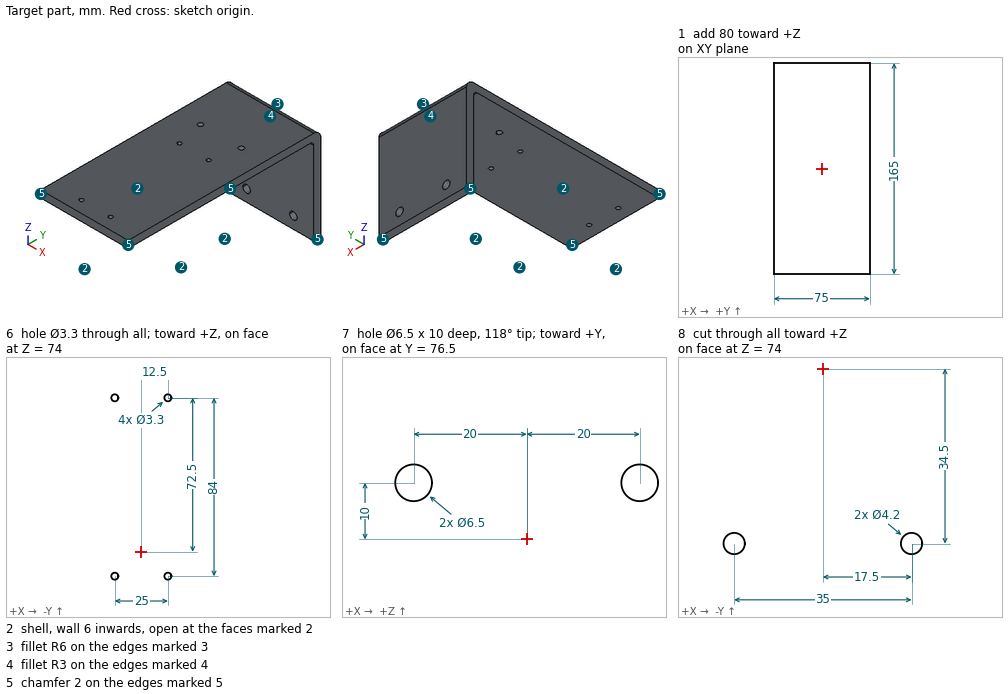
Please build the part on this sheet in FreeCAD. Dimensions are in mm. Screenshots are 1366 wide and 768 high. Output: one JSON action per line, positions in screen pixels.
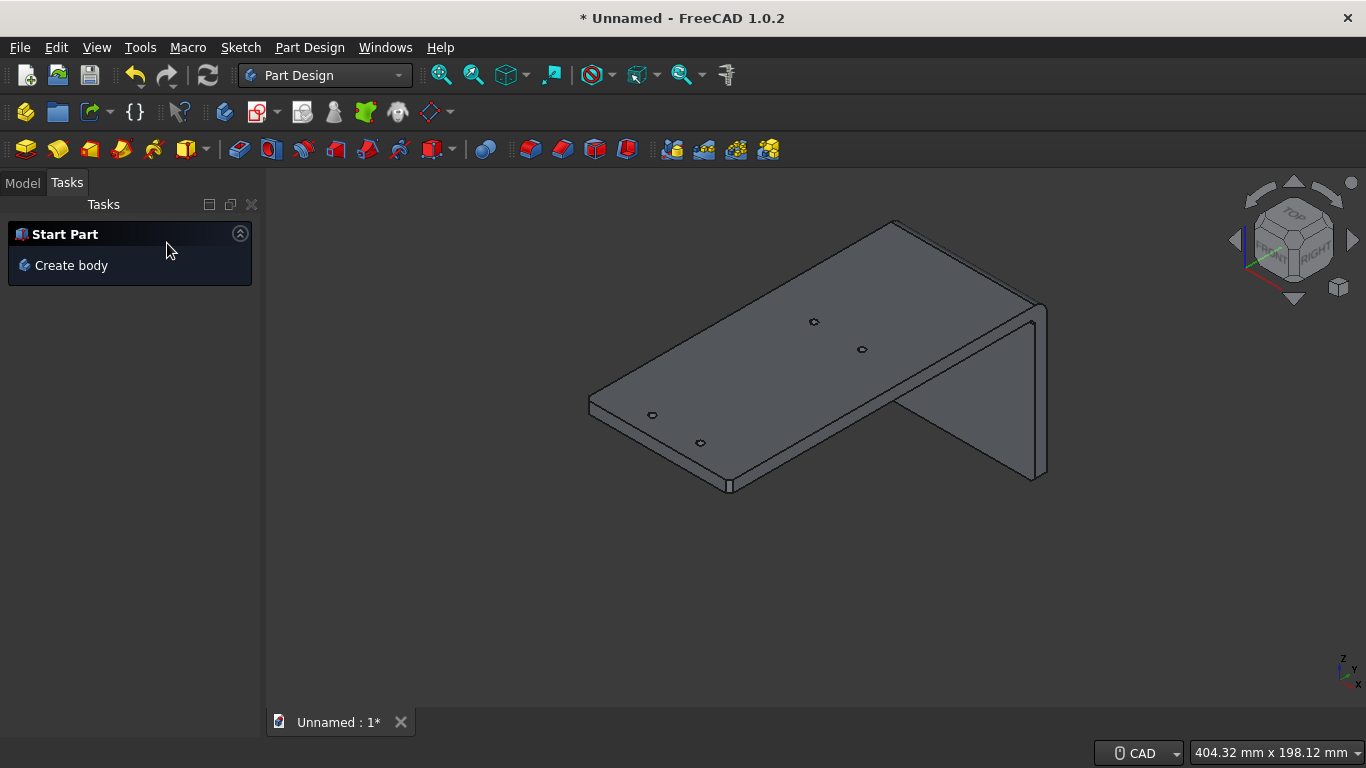
{"action": "left_click", "coordinate": [984, 373]}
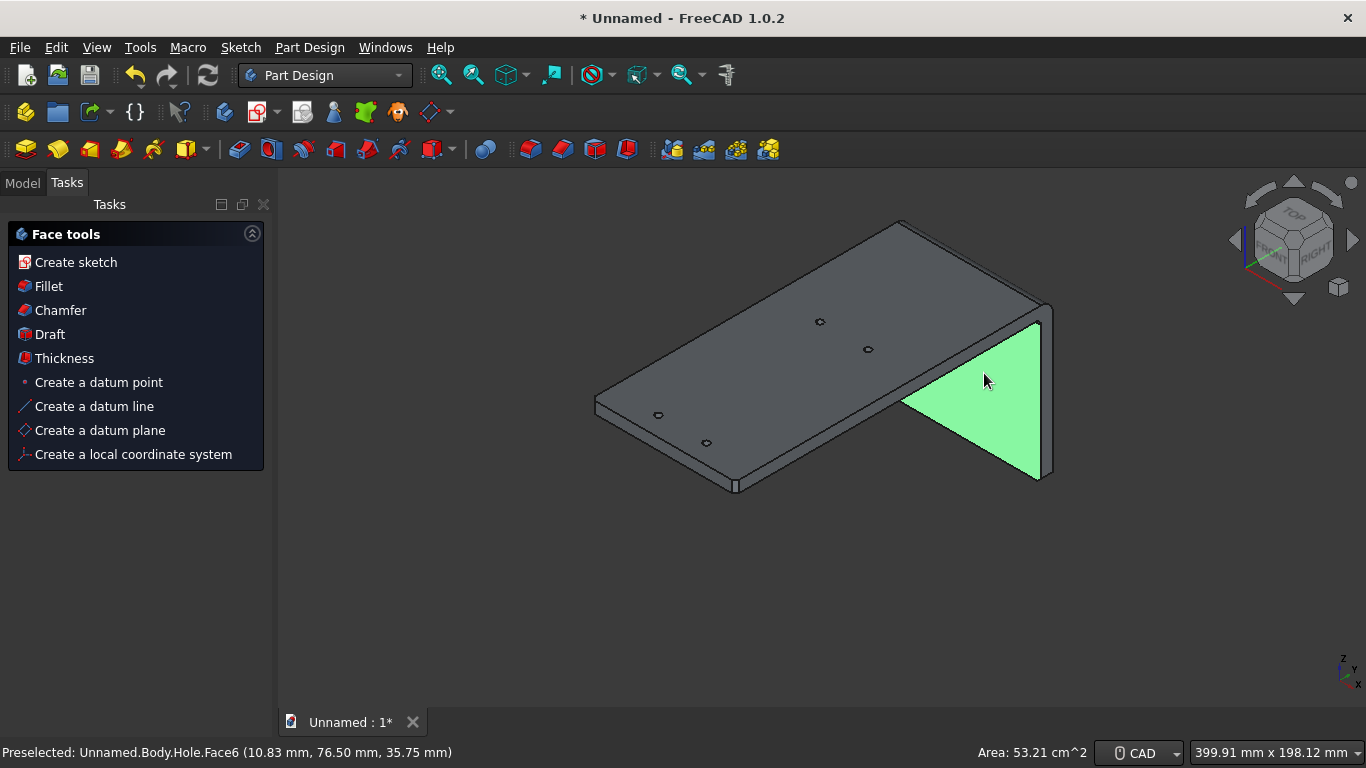
{"action": "left_click", "coordinate": [258, 112]}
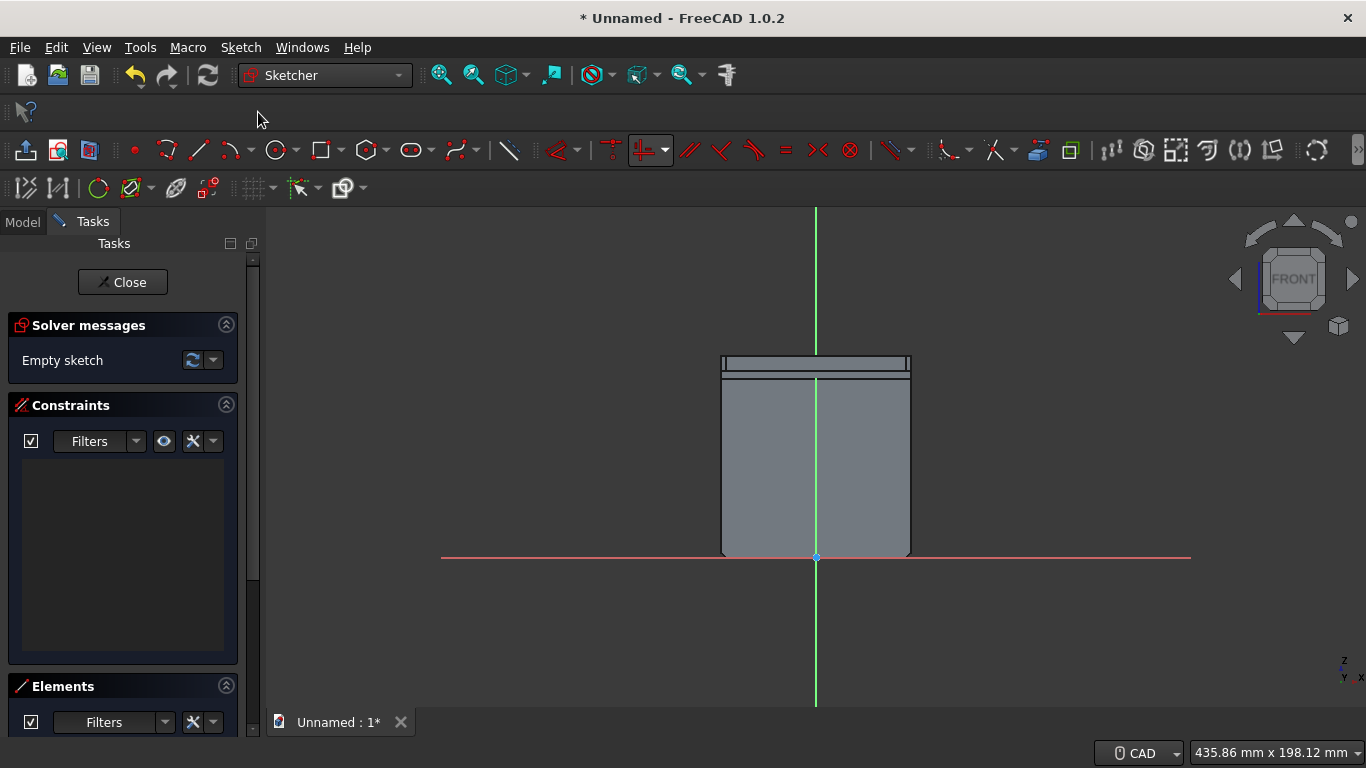
{"action": "scroll", "coordinate": [833, 563], "scroll_direction": "up", "scroll_amount": 8}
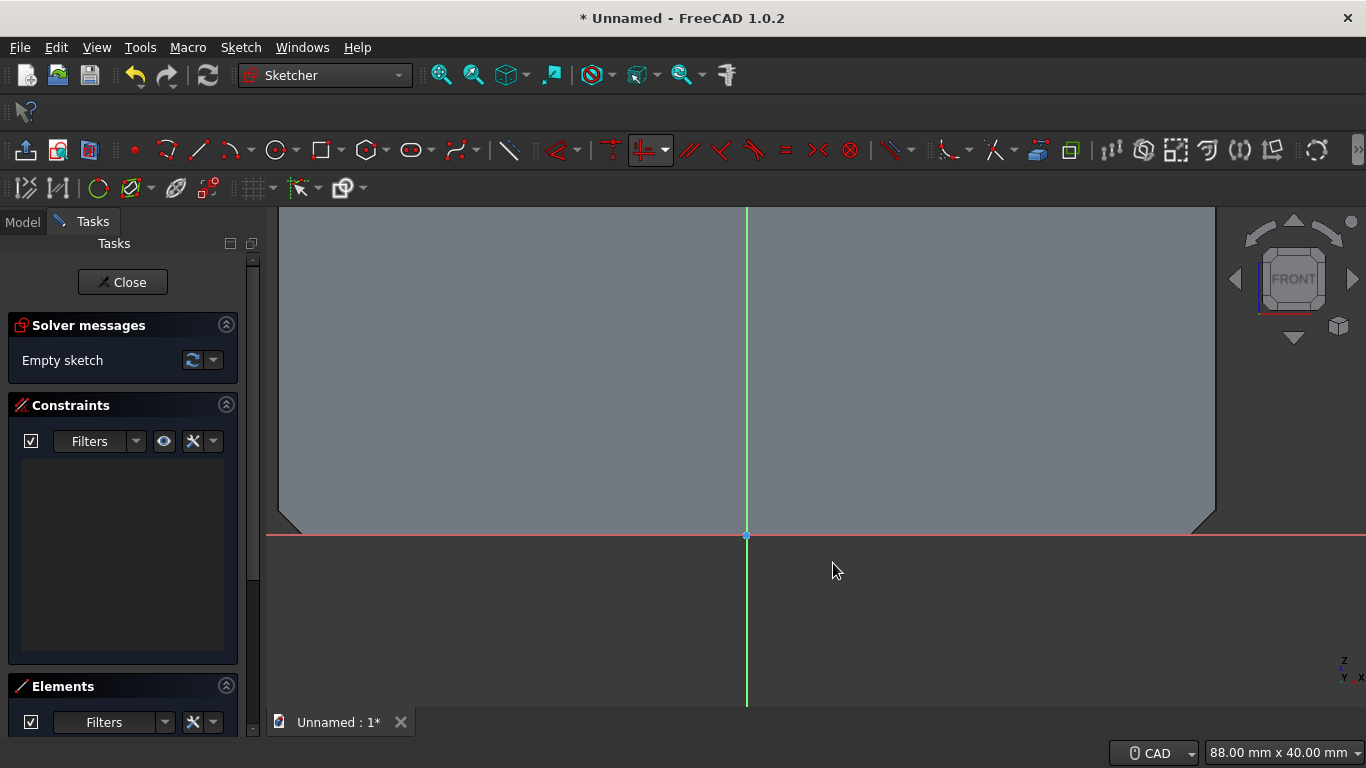
{"action": "left_click", "coordinate": [276, 150]}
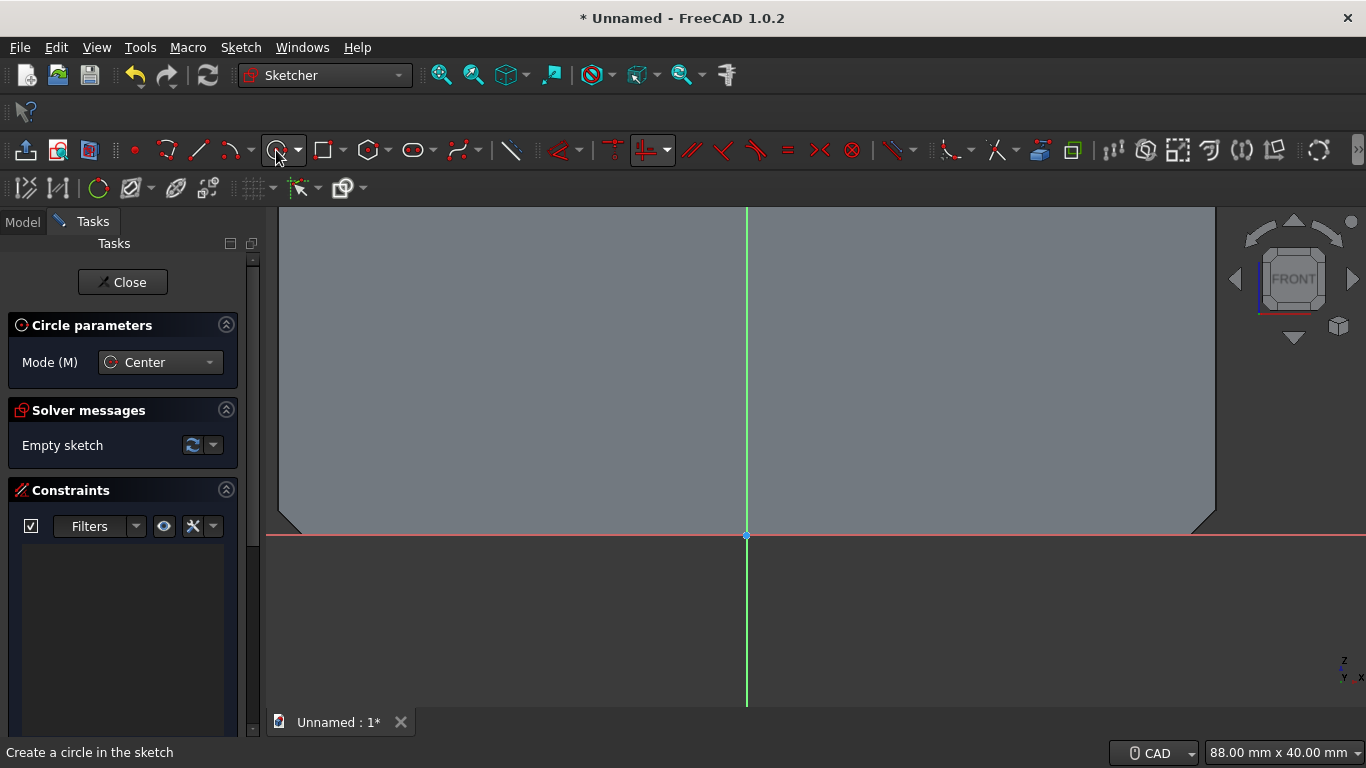
{"action": "left_click", "coordinate": [497, 410]}
{"action": "left_click", "coordinate": [525, 381]}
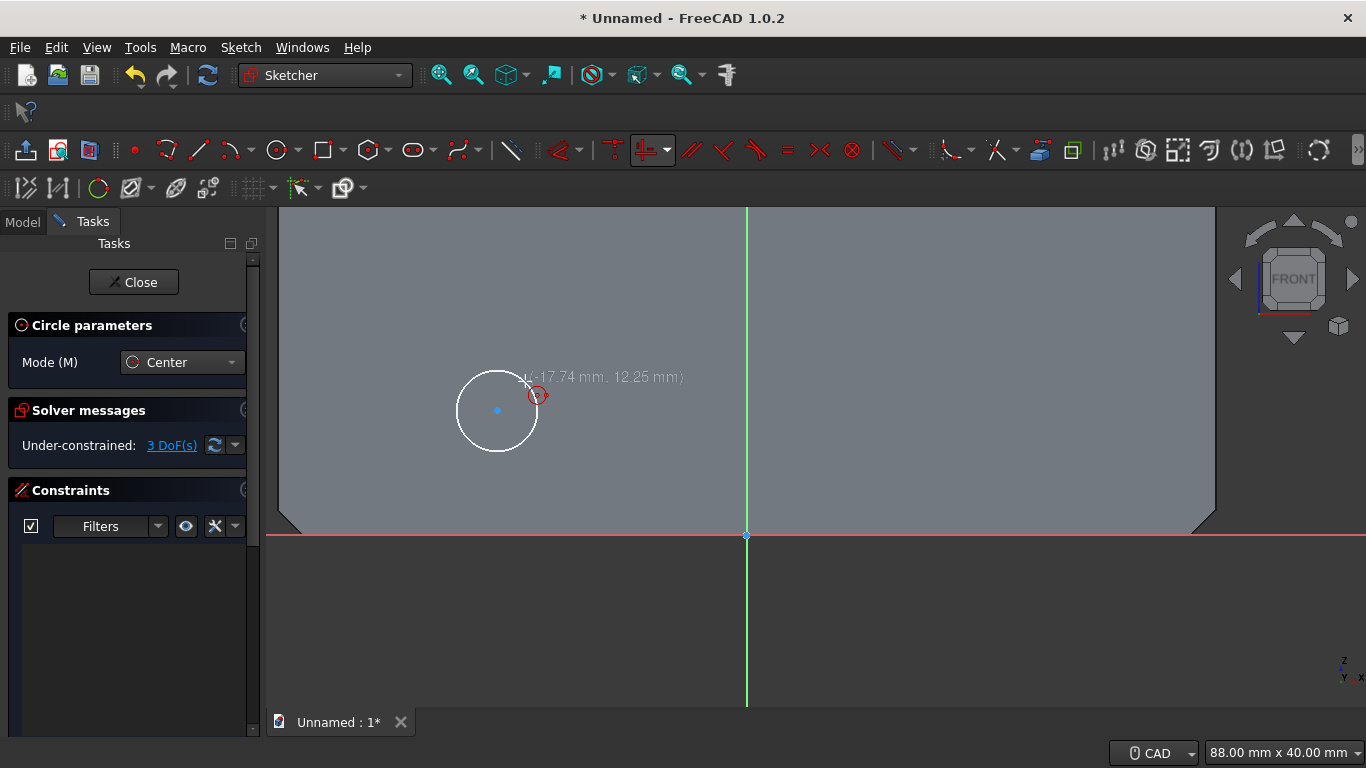
{"action": "left_click", "coordinate": [997, 410]}
{"action": "left_click", "coordinate": [1025, 381]}
{"action": "key", "text": "Escape"}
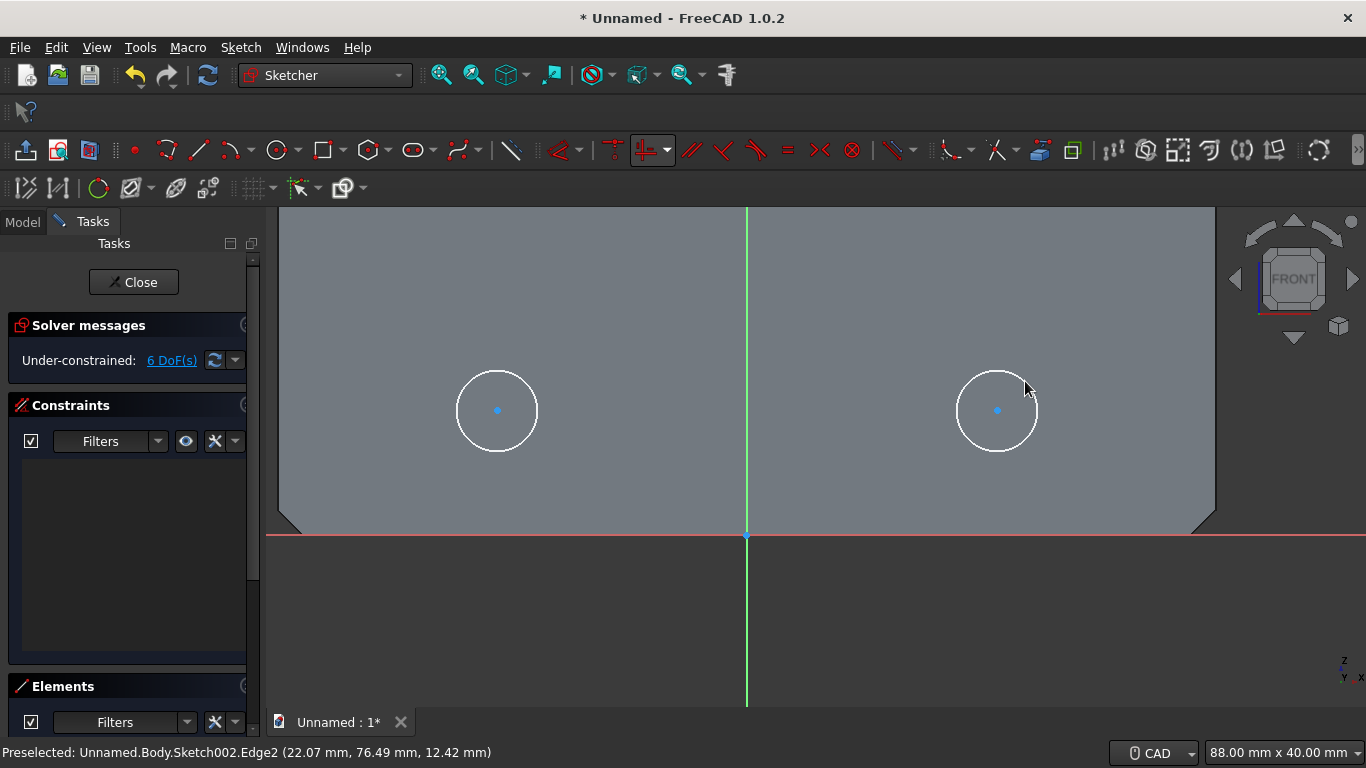
{"action": "left_click", "coordinate": [525, 382]}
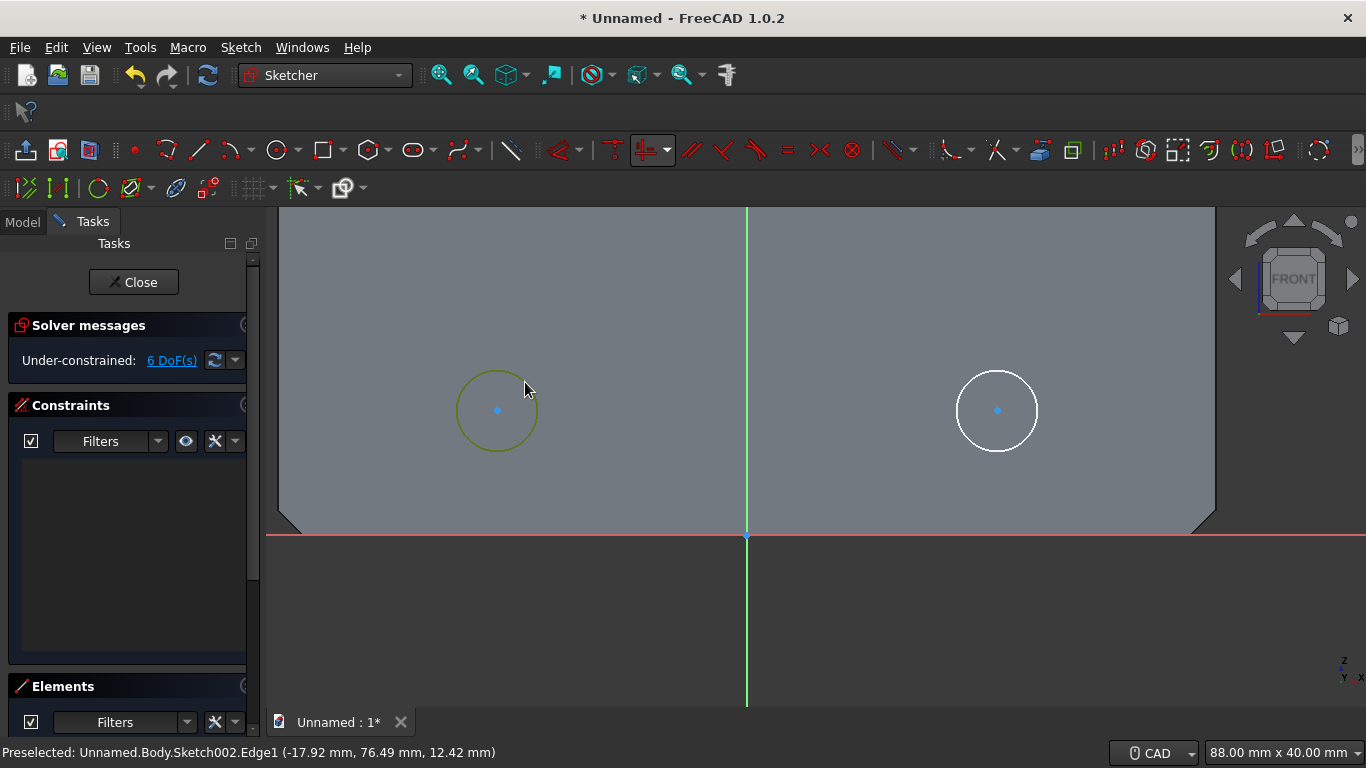
{"action": "left_click", "coordinate": [1025, 382]}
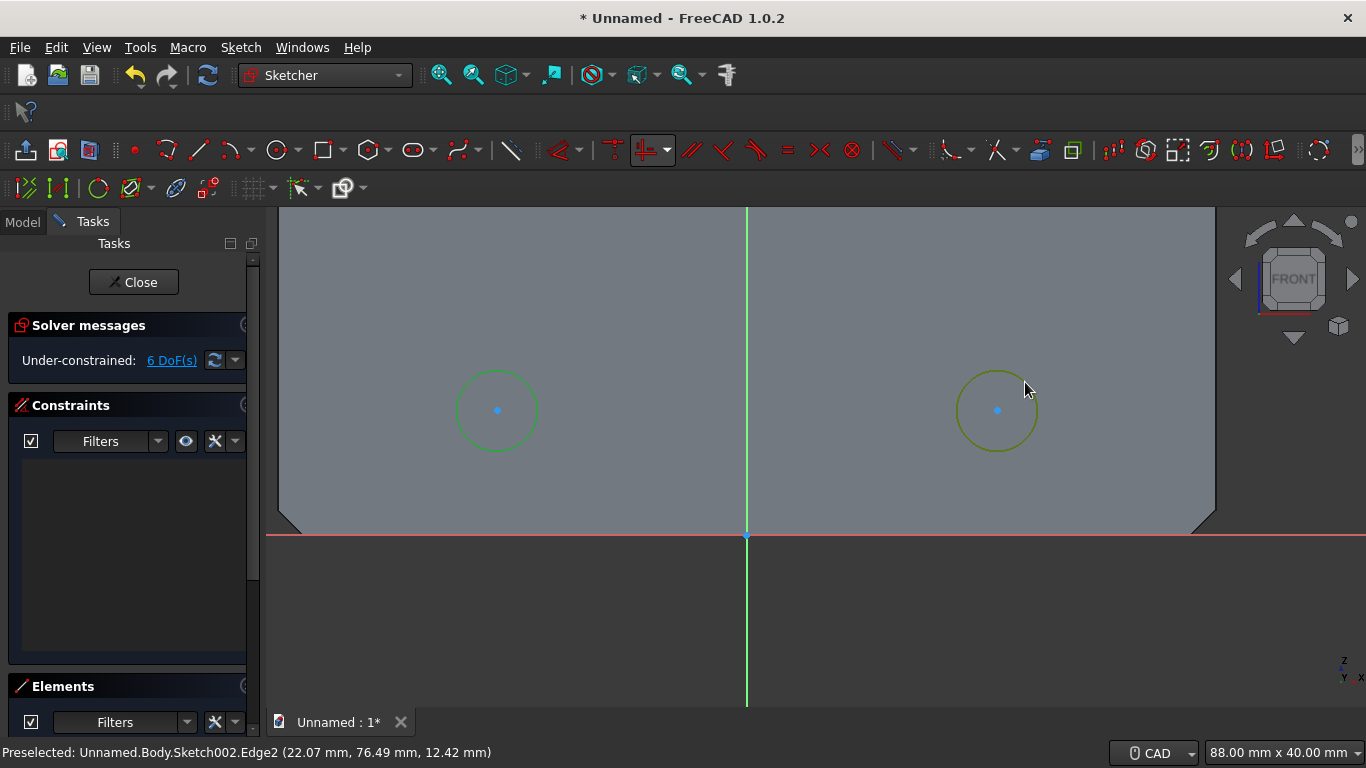
{"action": "left_click", "coordinate": [788, 150]}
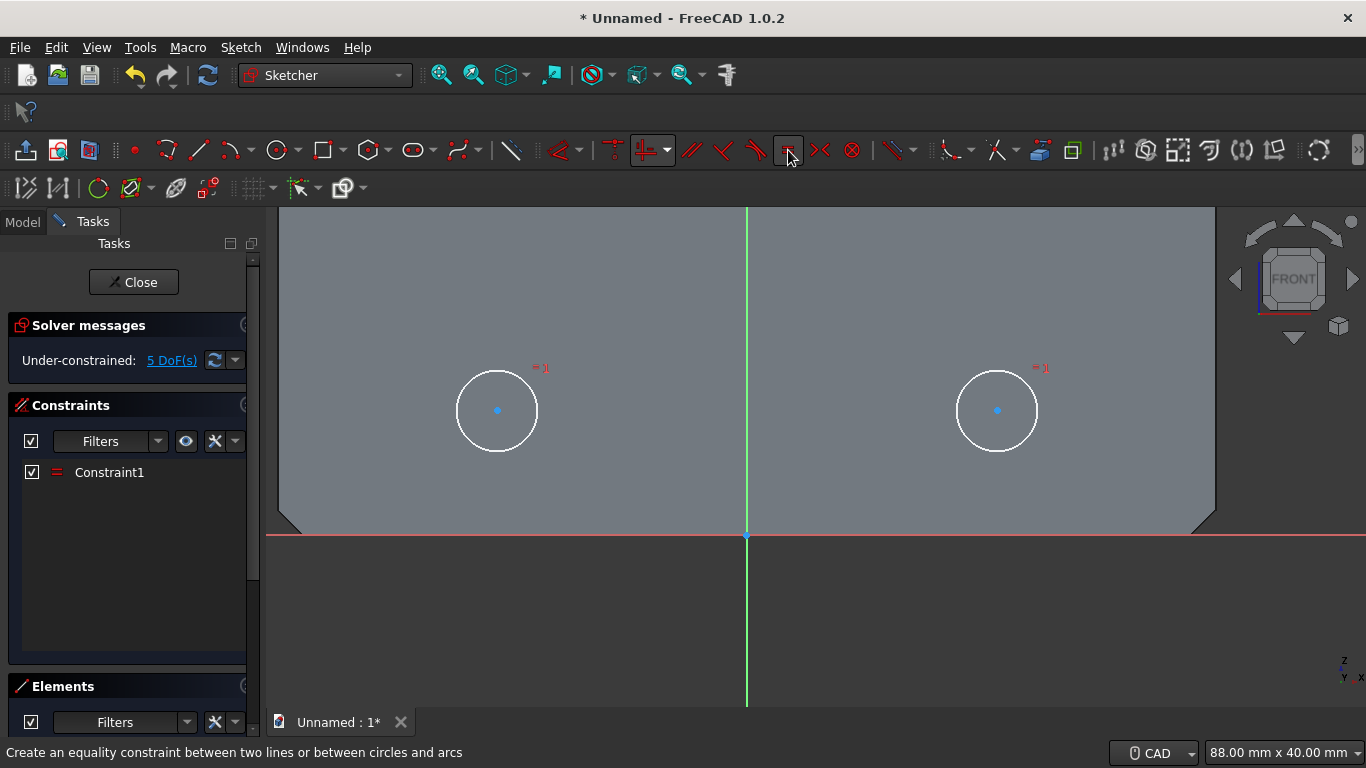
{"action": "left_click", "coordinate": [497, 411]}